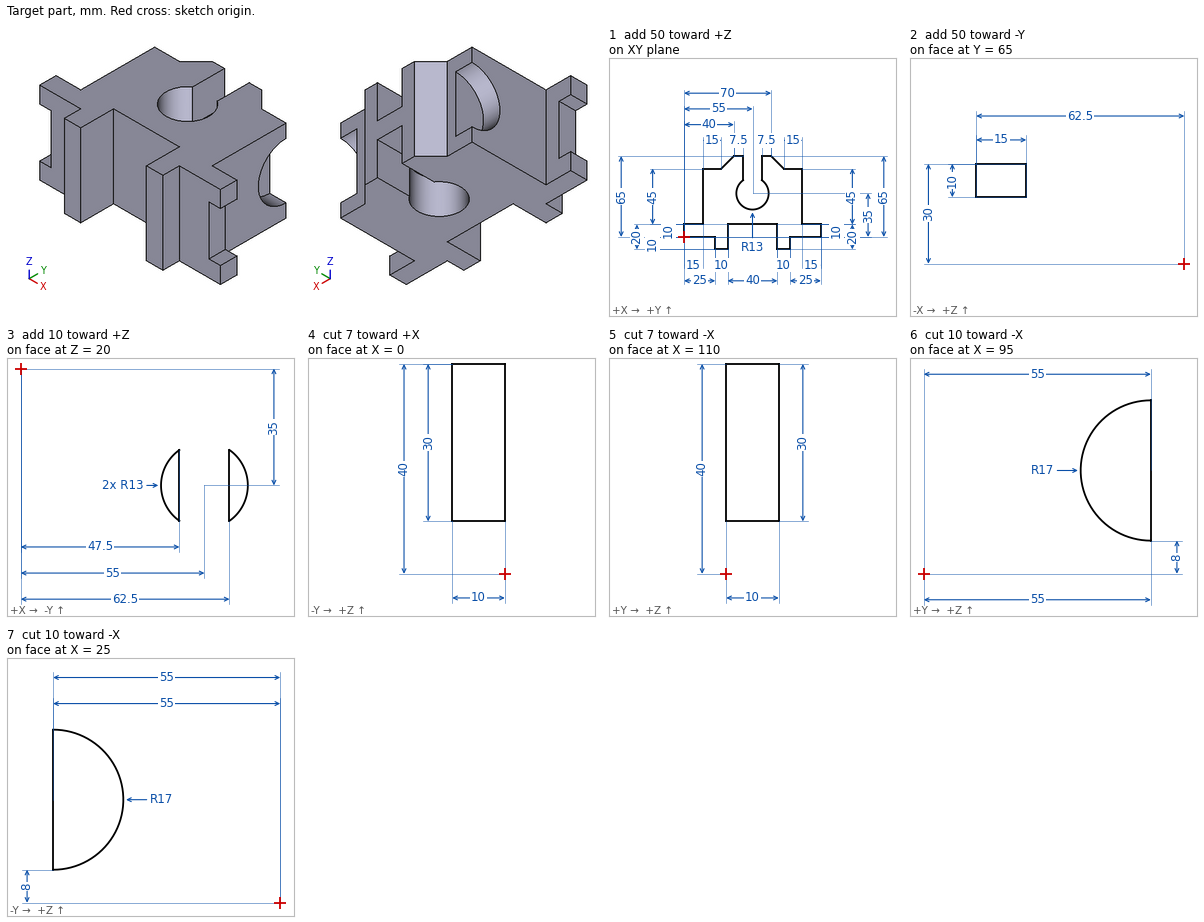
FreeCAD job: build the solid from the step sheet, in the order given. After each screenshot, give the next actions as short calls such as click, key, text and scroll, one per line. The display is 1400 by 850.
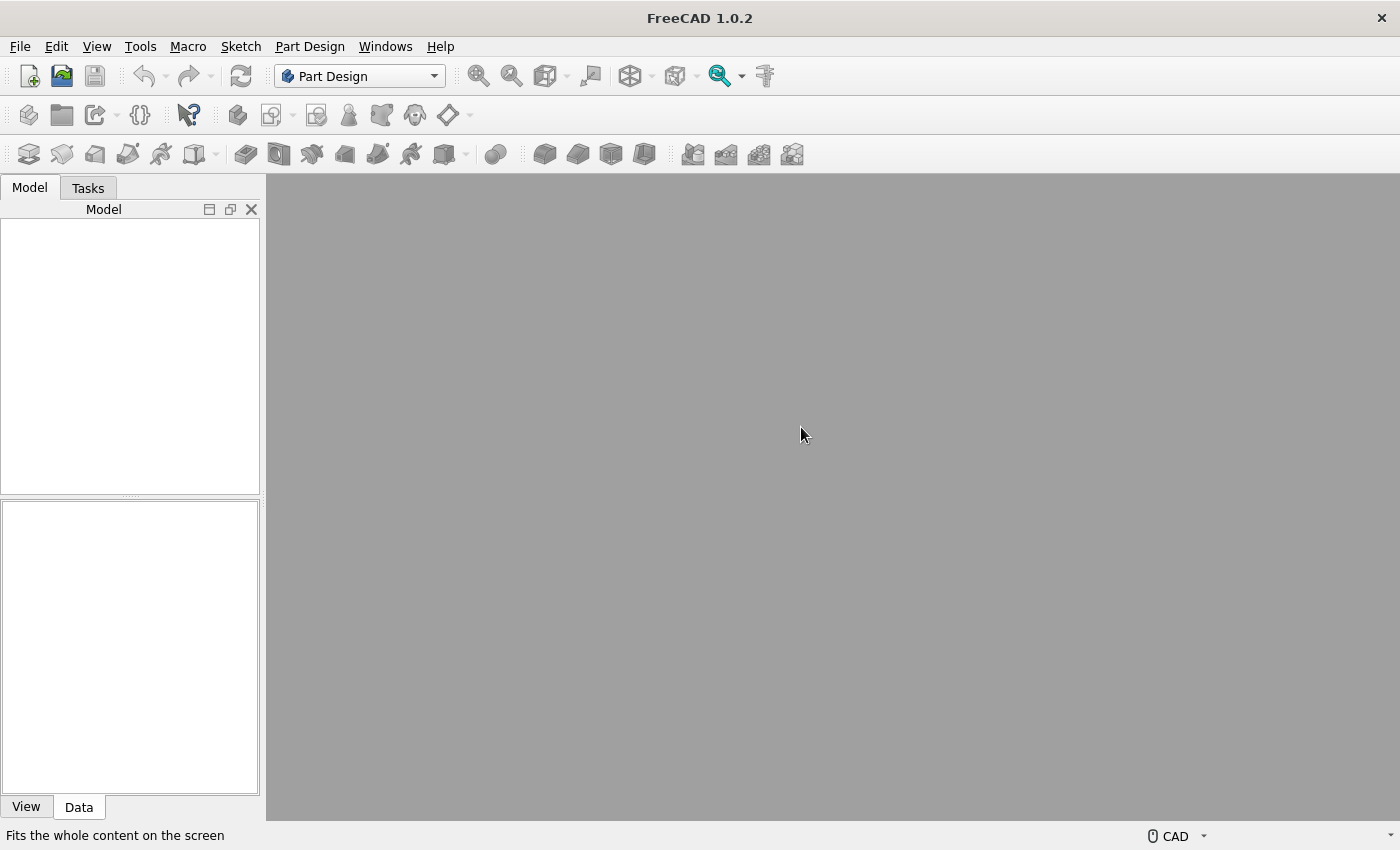
click(29, 76)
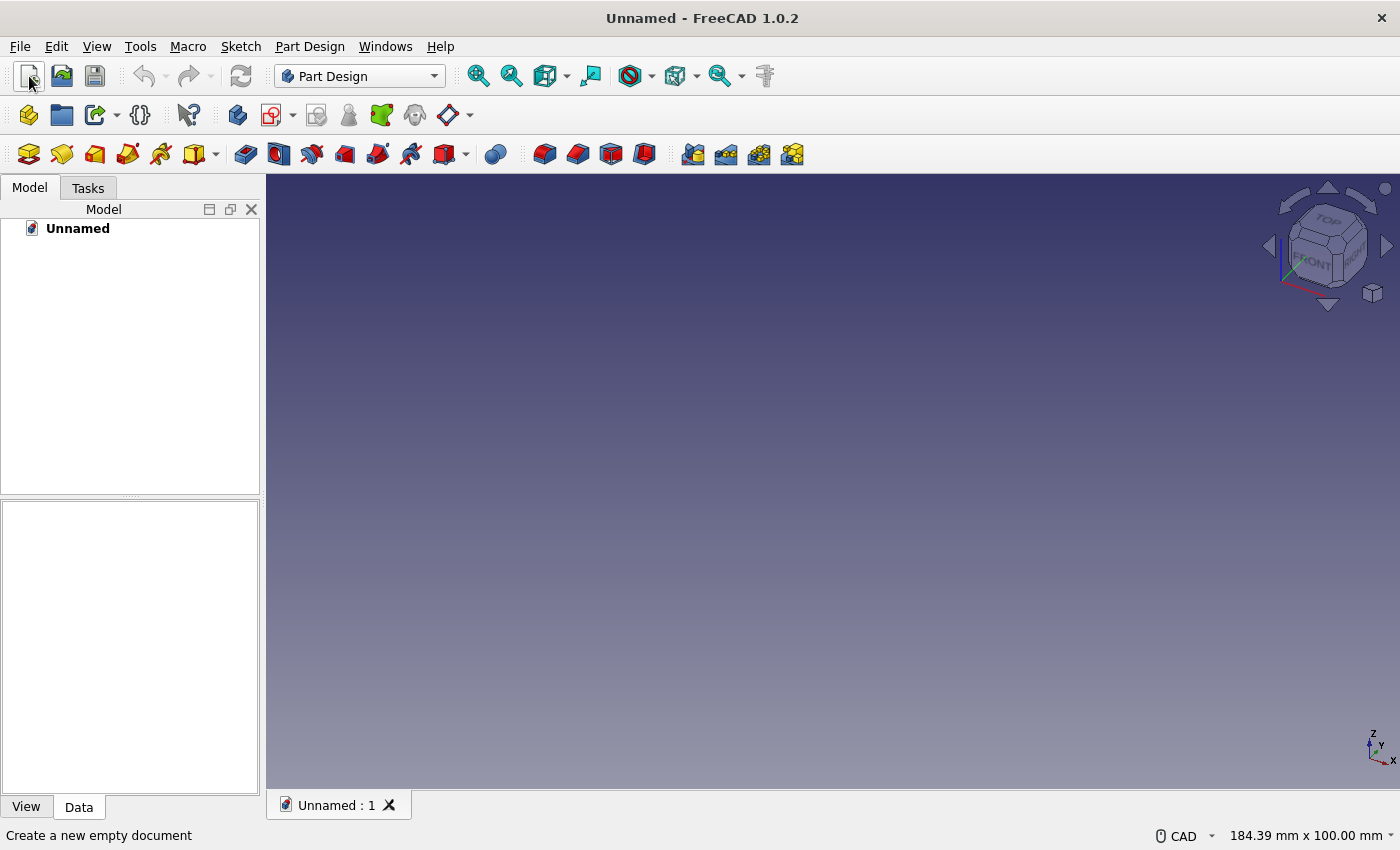
click(270, 116)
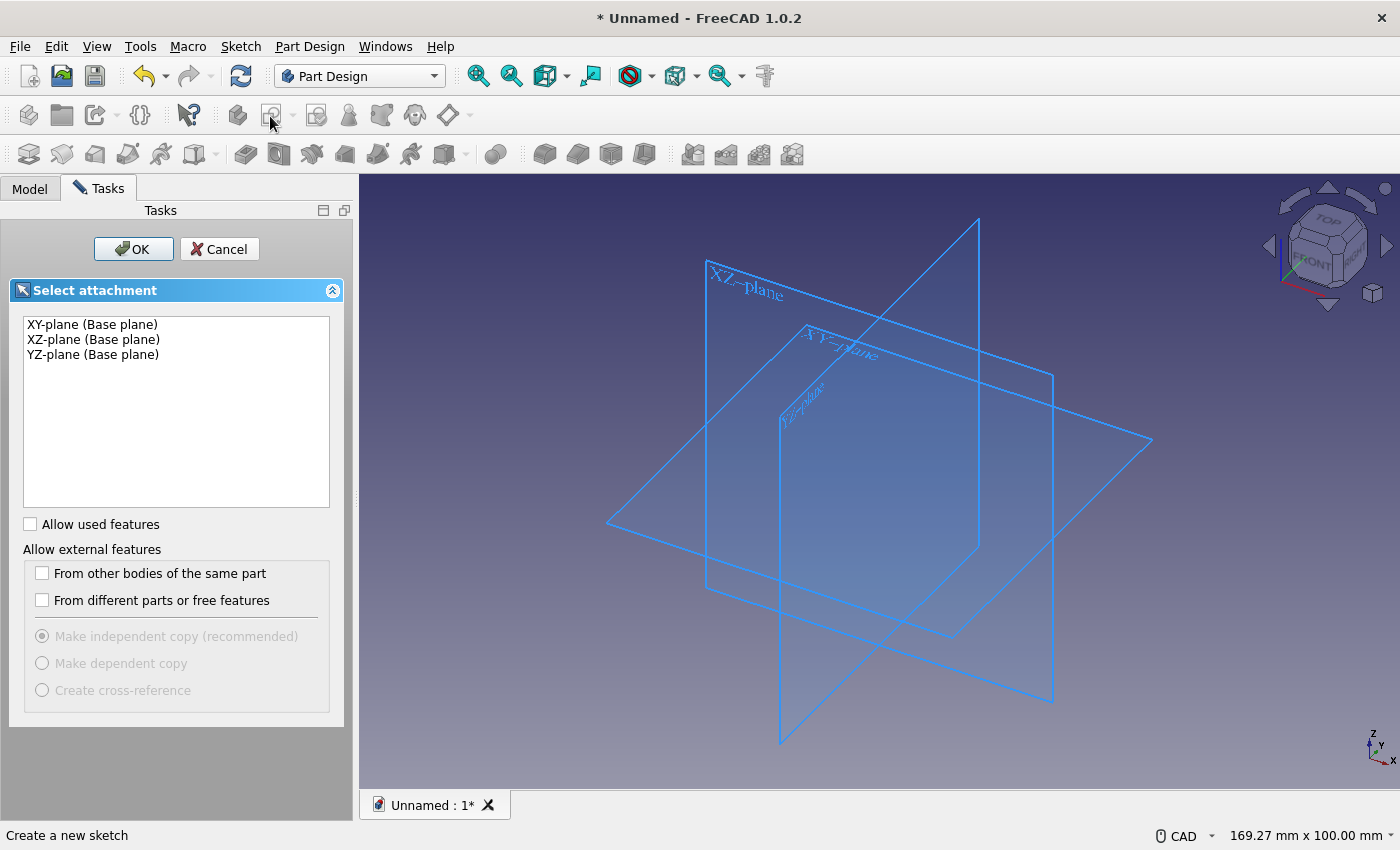
click(84, 324)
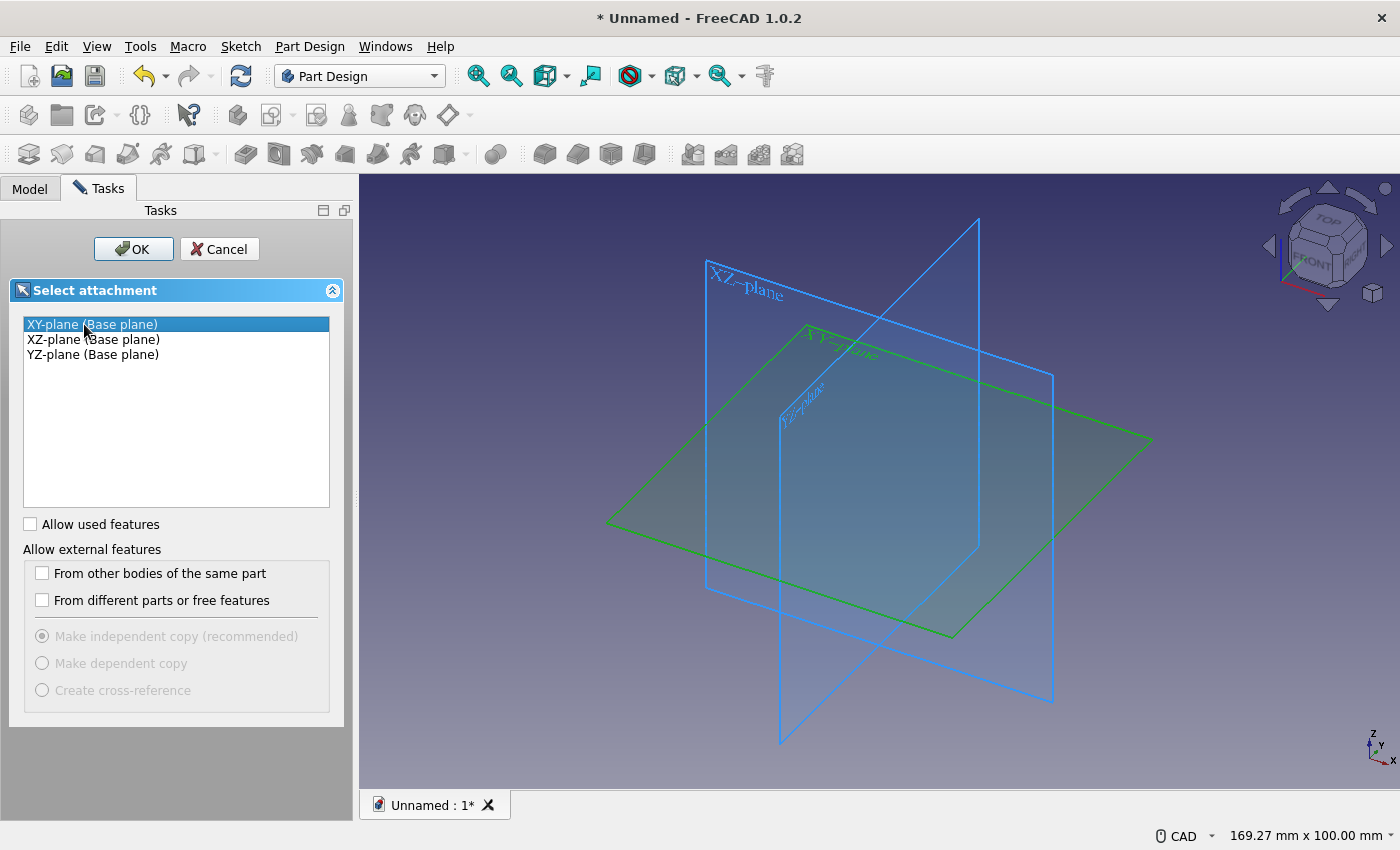
click(134, 249)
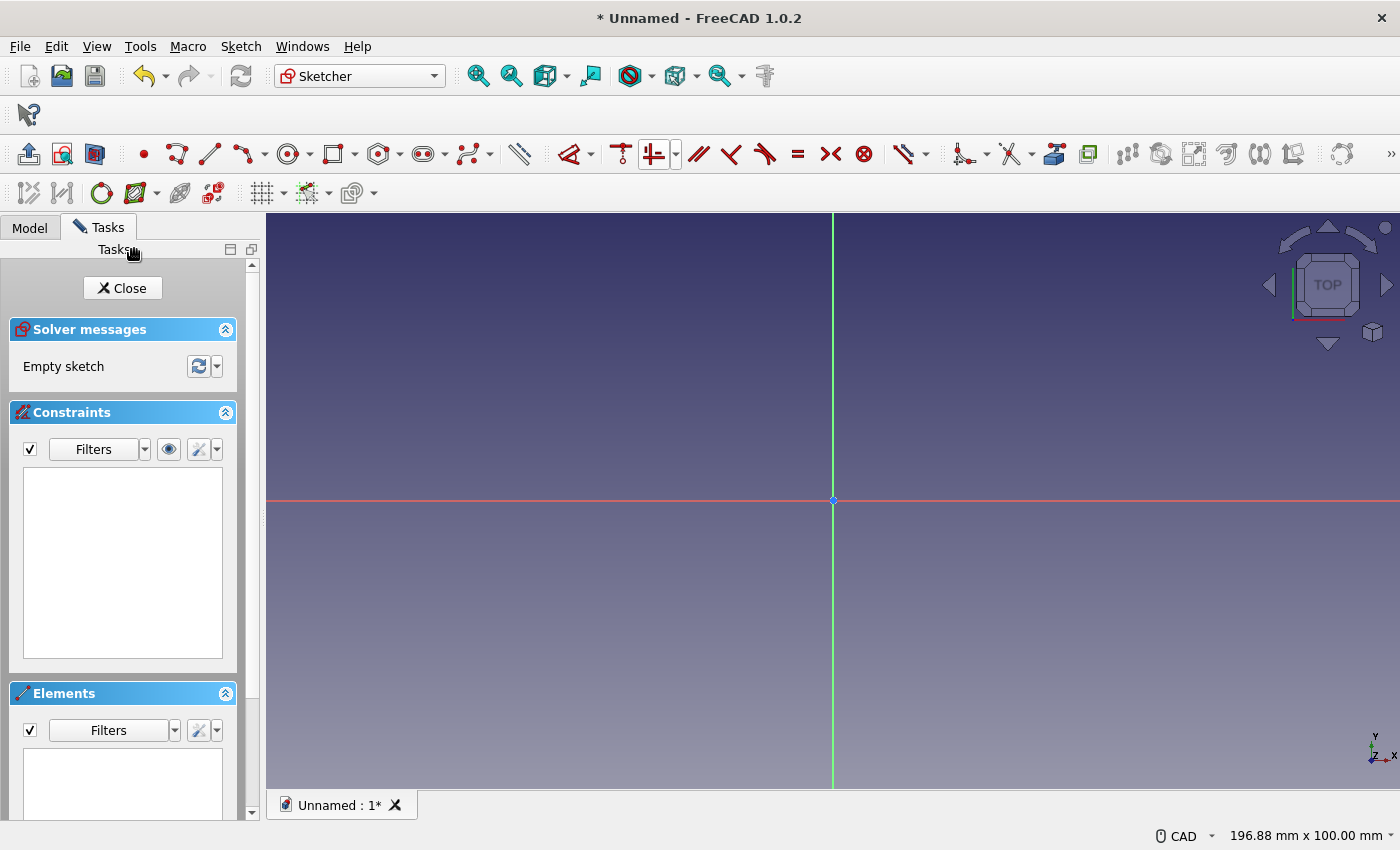
scroll(294, 761, down, 2)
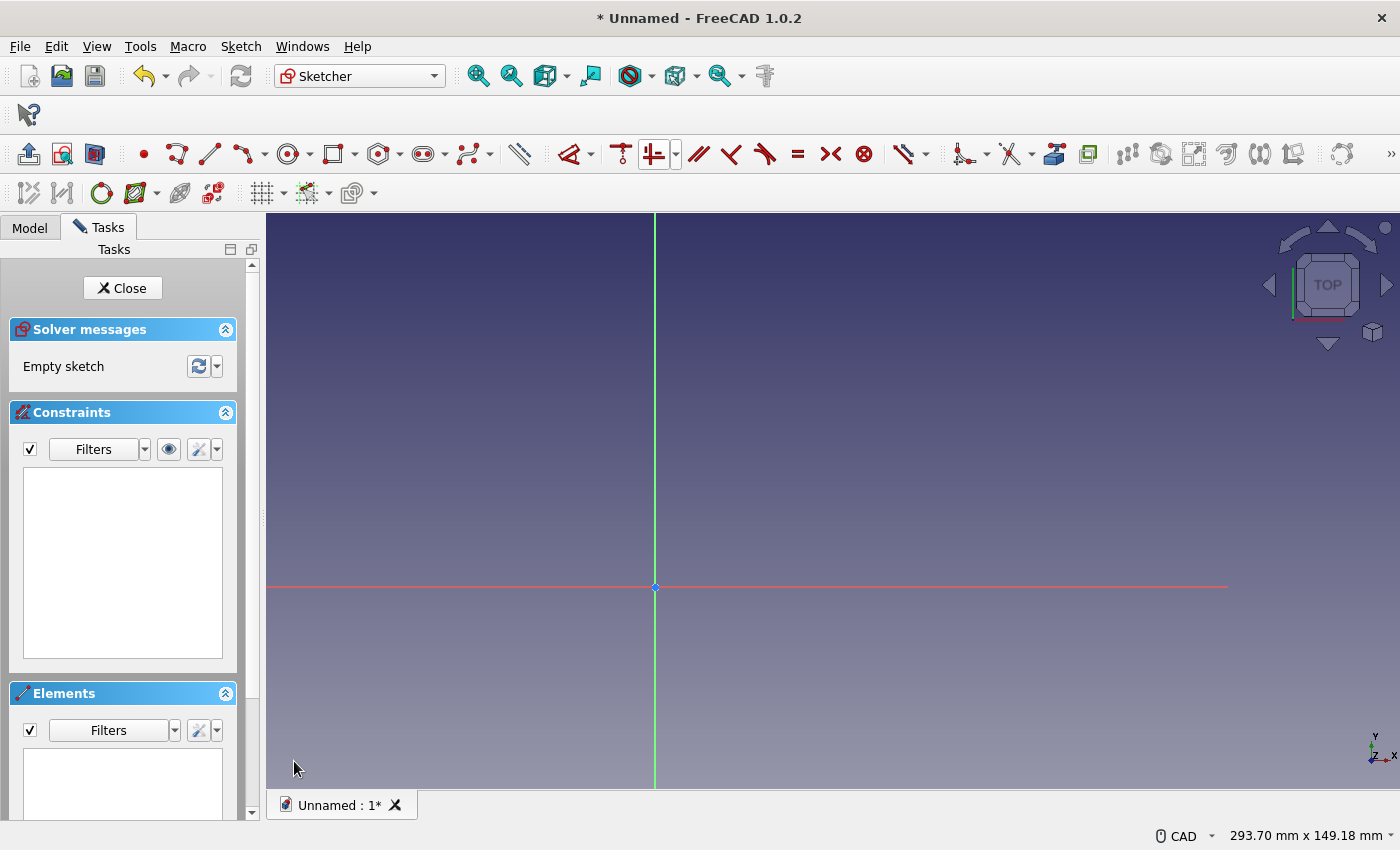
click(177, 154)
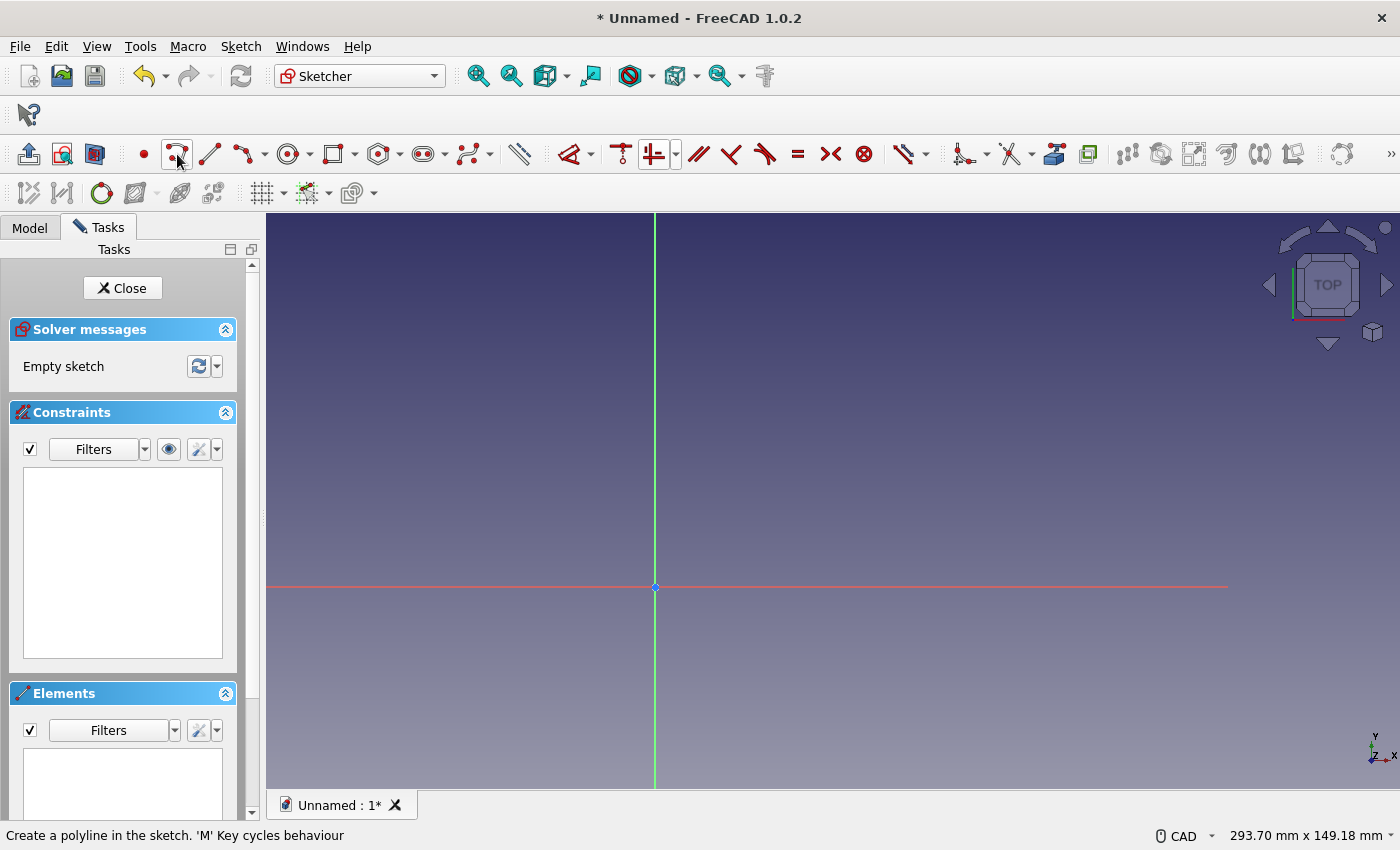
click(839, 411)
click(839, 336)
click(810, 336)
click(771, 375)
click(713, 375)
click(713, 548)
click(655, 548)
click(655, 587)
click(752, 578)
click(752, 626)
click(790, 626)
click(790, 548)
click(945, 548)
click(945, 626)
click(983, 626)
click(983, 587)
click(1080, 578)
click(1080, 548)
click(1022, 548)
click(1022, 375)
click(964, 375)
click(926, 336)
click(897, 336)
click(897, 411)
right_click(897, 411)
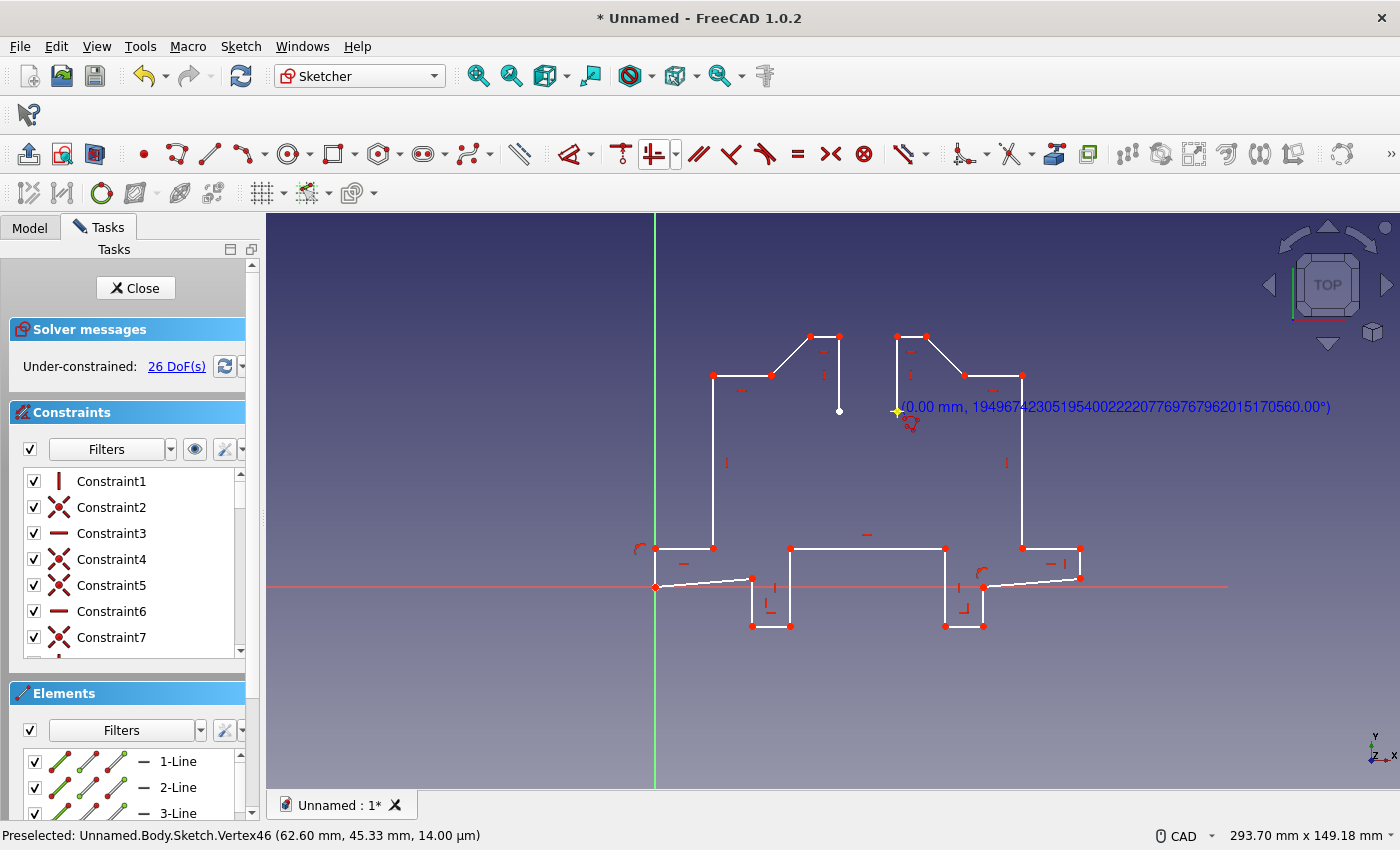
click(242, 154)